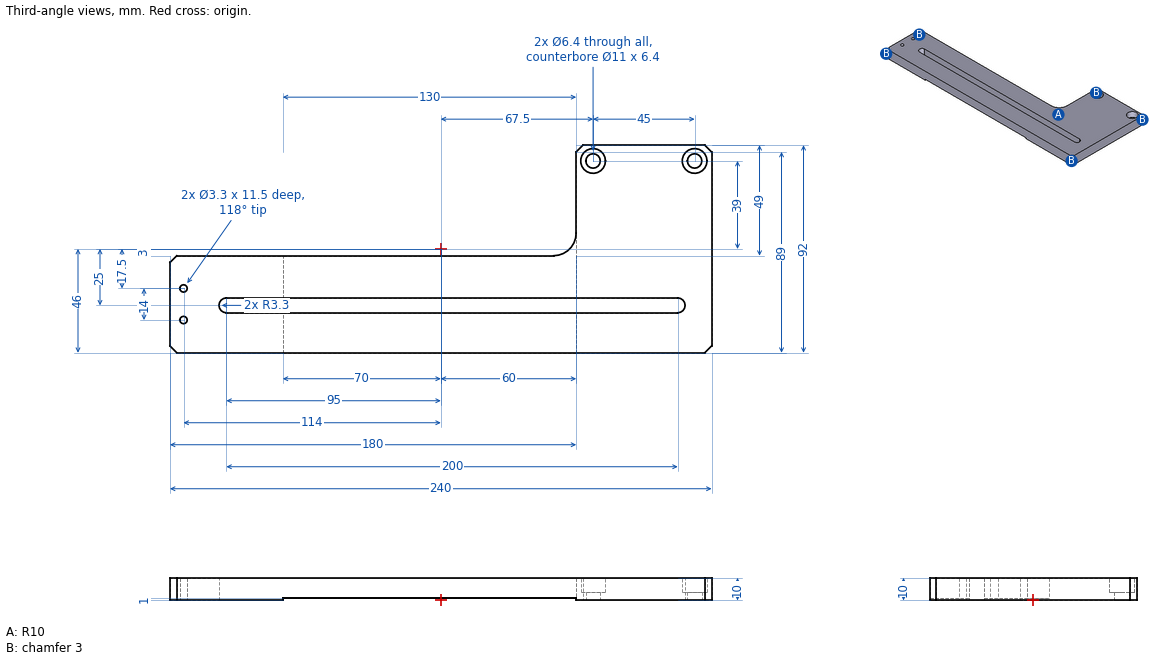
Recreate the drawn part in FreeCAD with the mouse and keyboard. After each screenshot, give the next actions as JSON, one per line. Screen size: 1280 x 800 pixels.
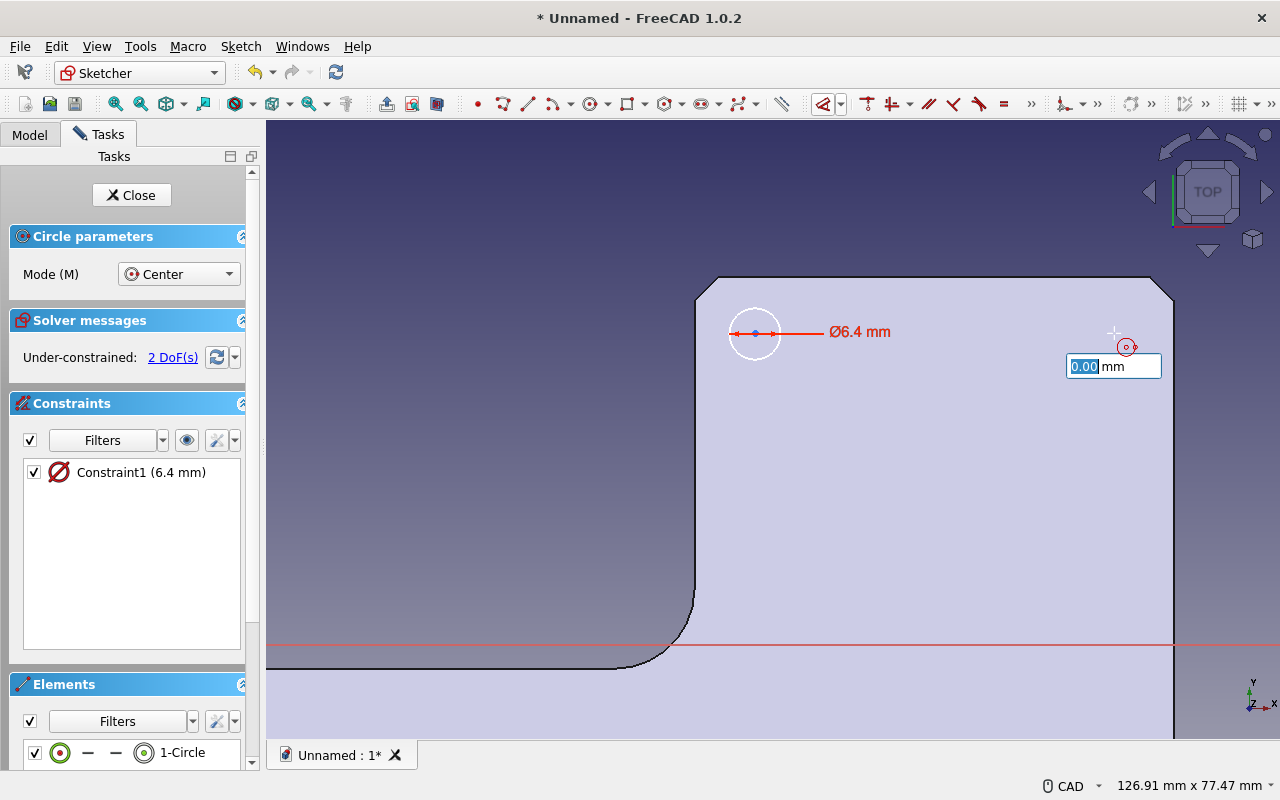
{"action": "scroll", "coordinate": [760, 335], "scroll_direction": "down", "scroll_amount": 2}
{"action": "mouse_move", "coordinate": [1010, 322]}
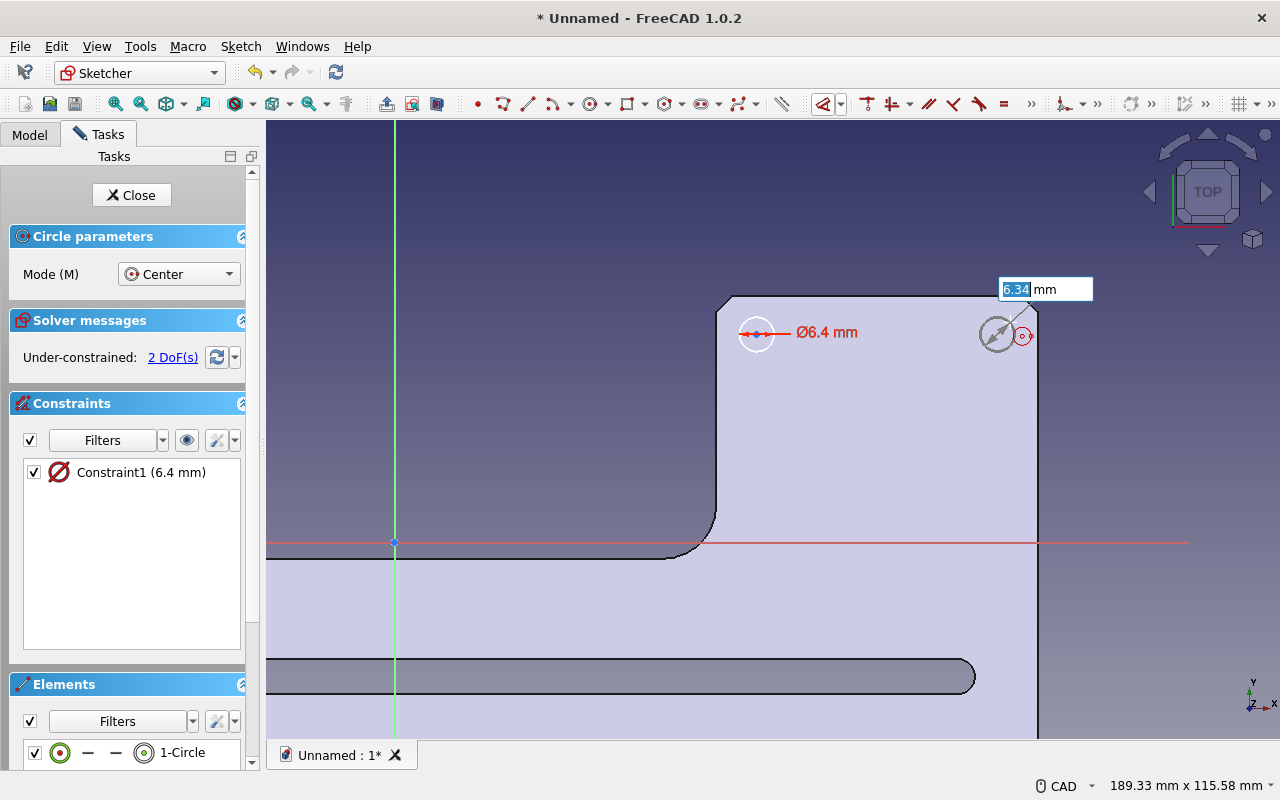
{"action": "type", "text": "6.4"}
{"action": "key", "text": "Return"}
{"action": "key", "text": "Escape"}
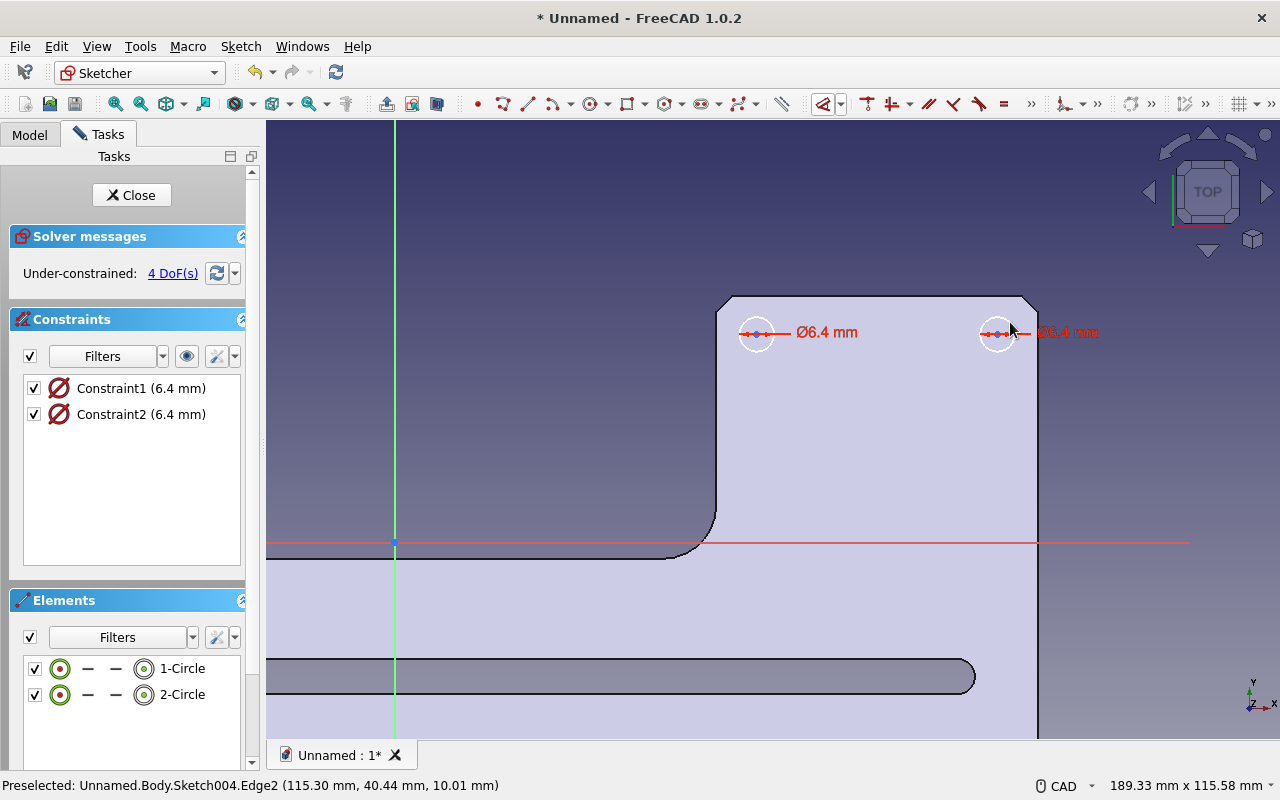
{"action": "left_click", "coordinate": [757, 334]}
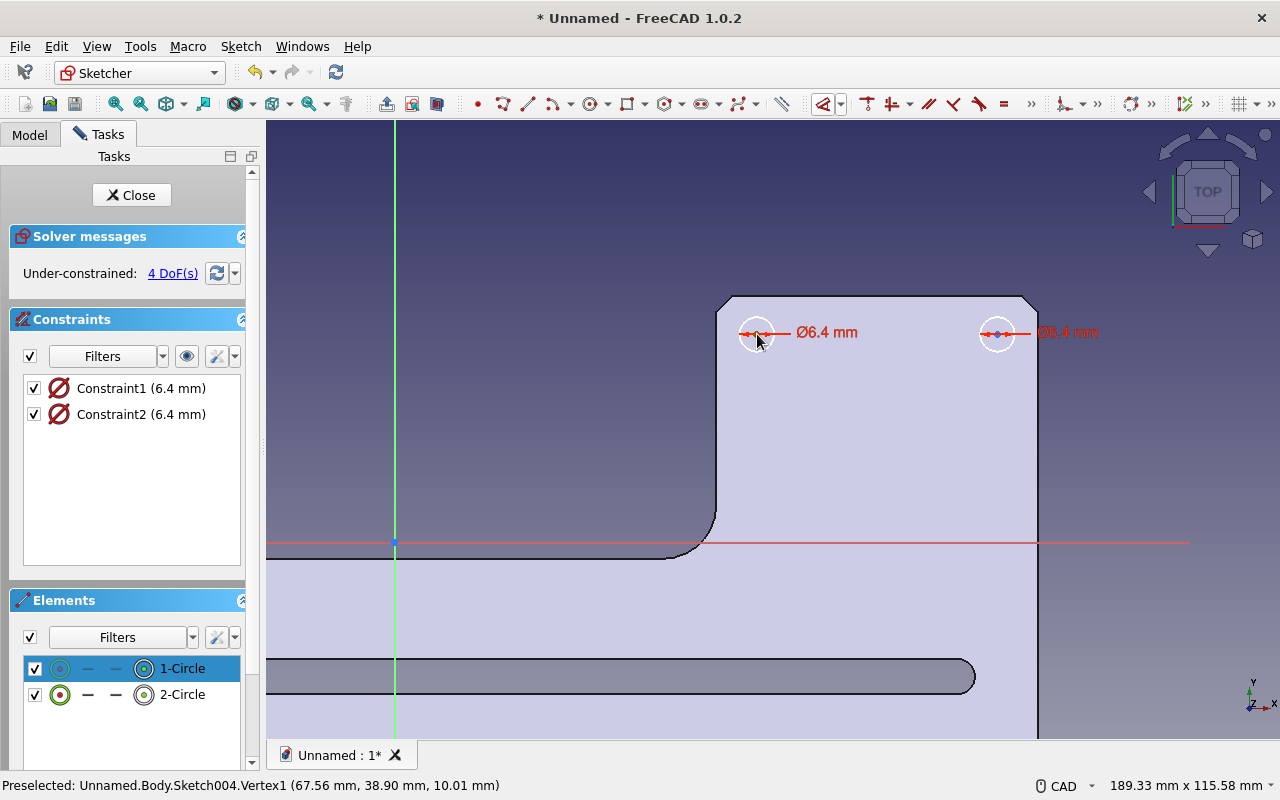
{"action": "key", "text": "i"}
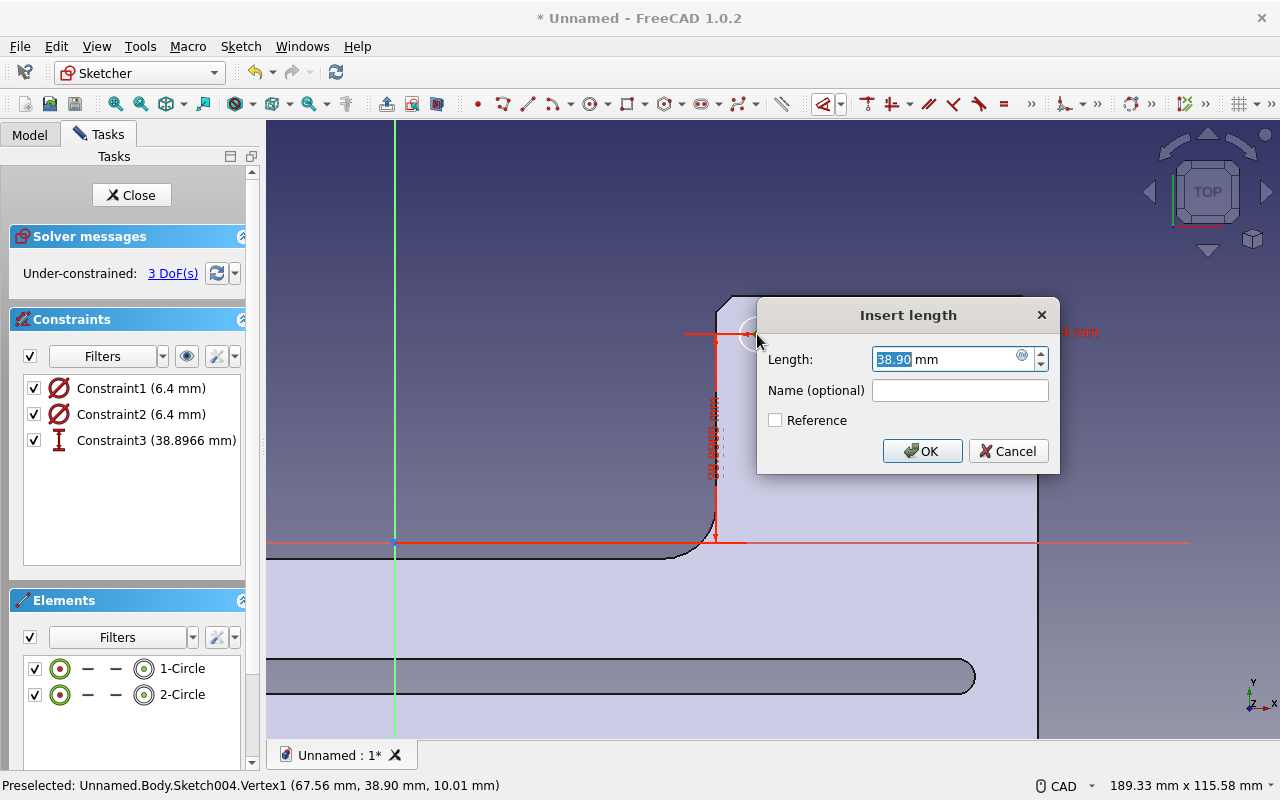
{"action": "type", "text": "39"}
{"action": "key", "text": "Return"}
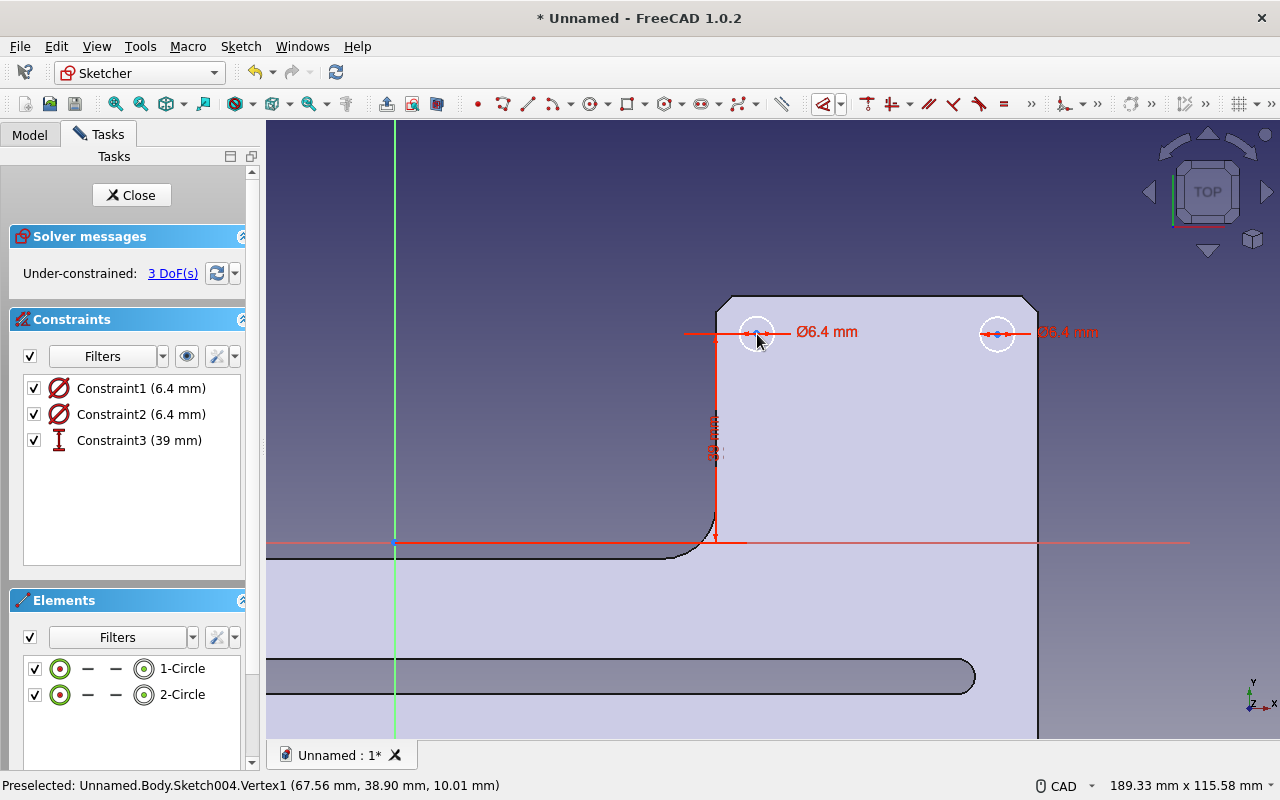
{"action": "left_click", "coordinate": [997, 334]}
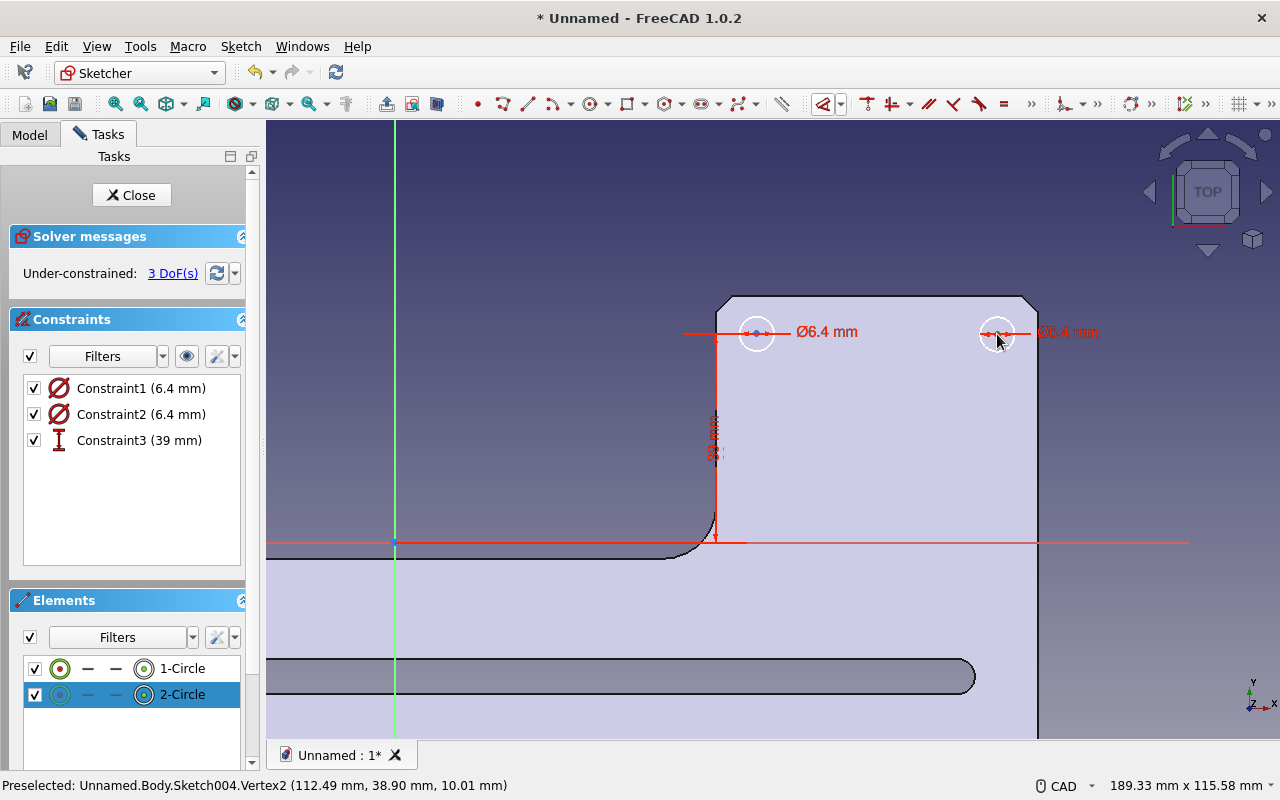
{"action": "key", "text": "i"}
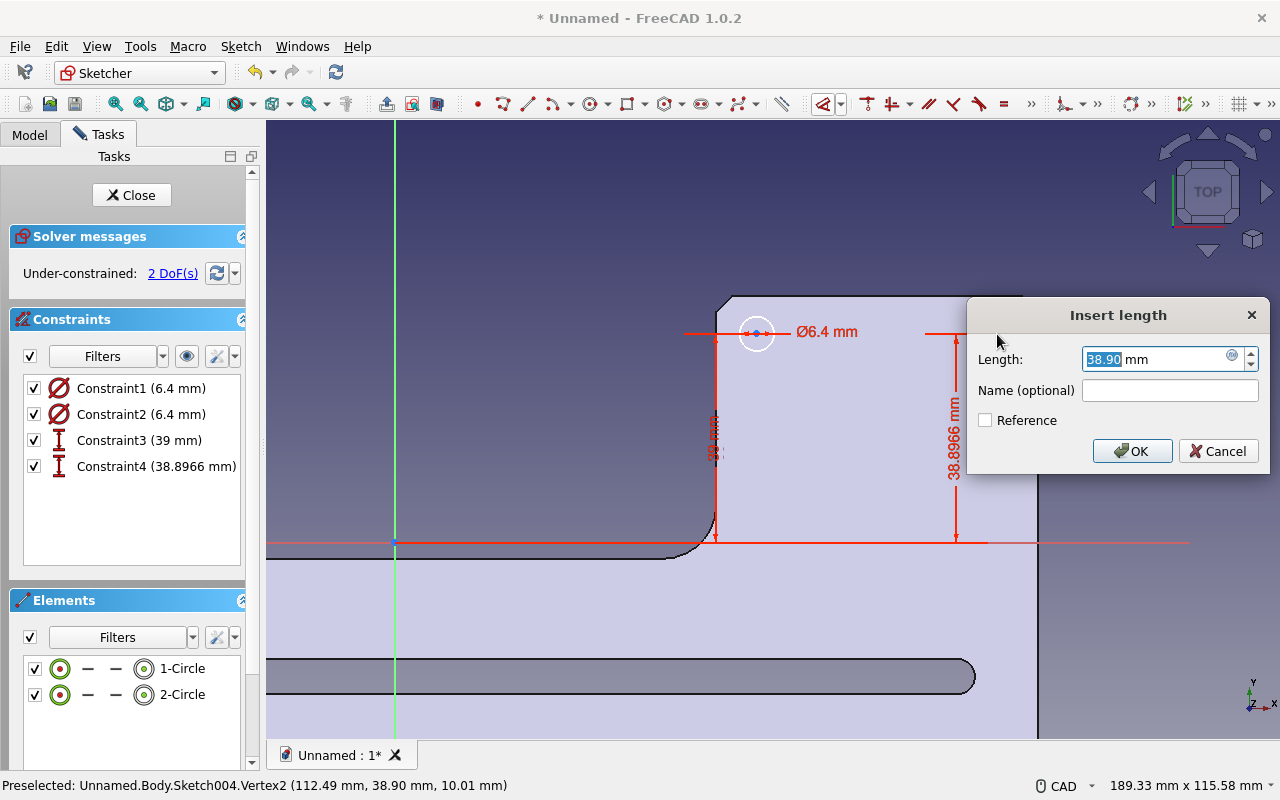
{"action": "type", "text": "39"}
{"action": "key", "text": "Return"}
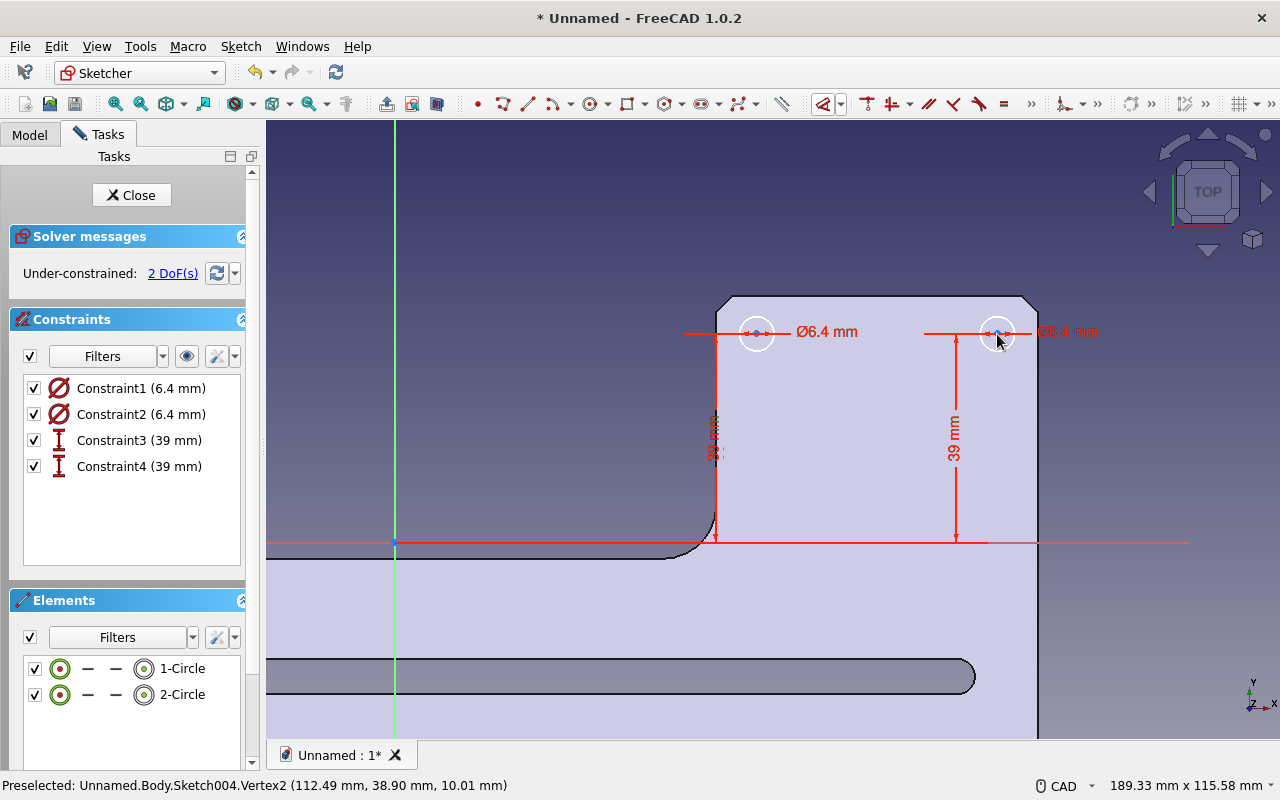
{"action": "left_click", "coordinate": [757, 334]}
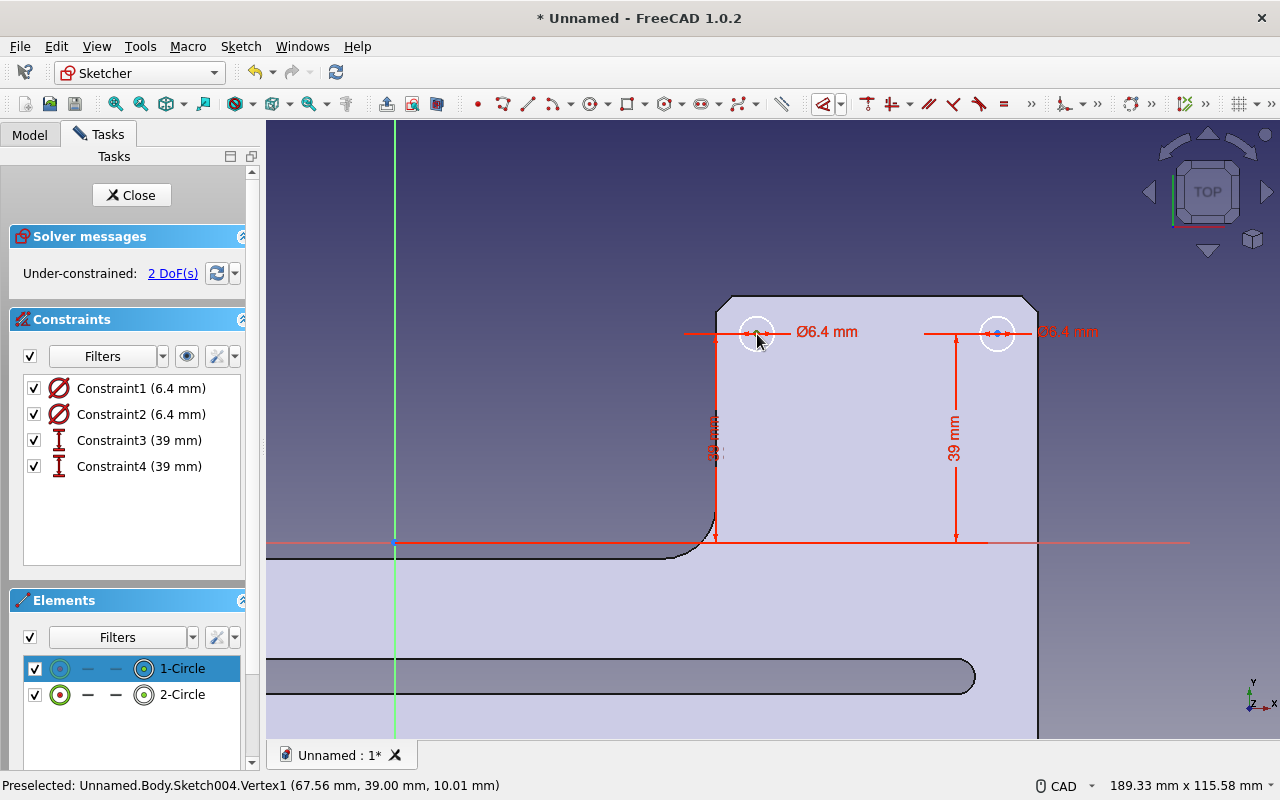
{"action": "left_click", "coordinate": [997, 334]}